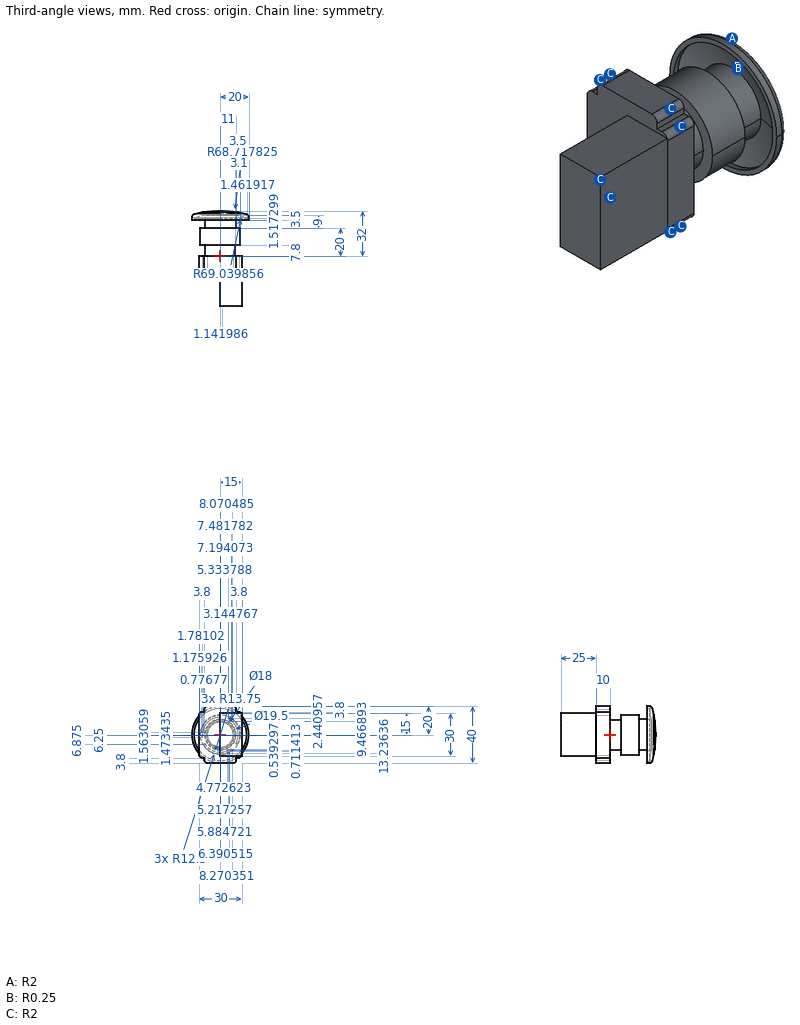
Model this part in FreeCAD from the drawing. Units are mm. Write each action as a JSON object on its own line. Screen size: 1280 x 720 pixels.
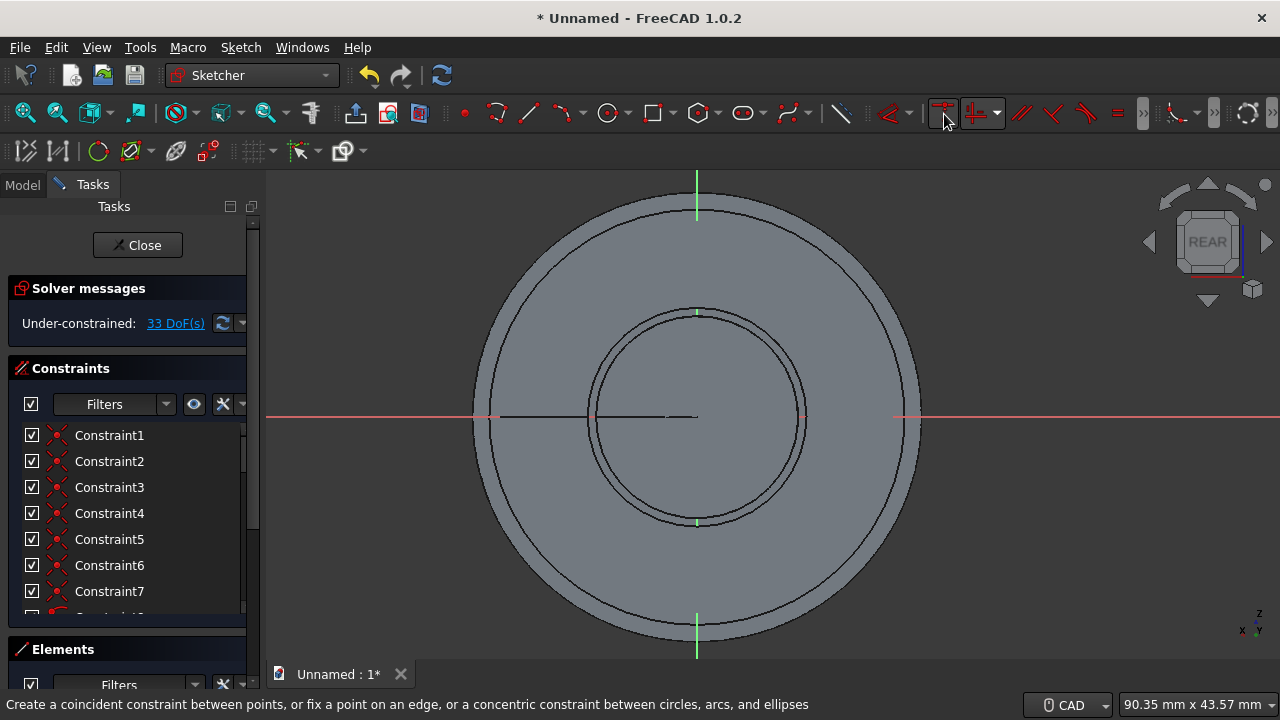
{"action": "left_click_drag", "start_coordinate": [687, 407], "coordinate": [707, 428]}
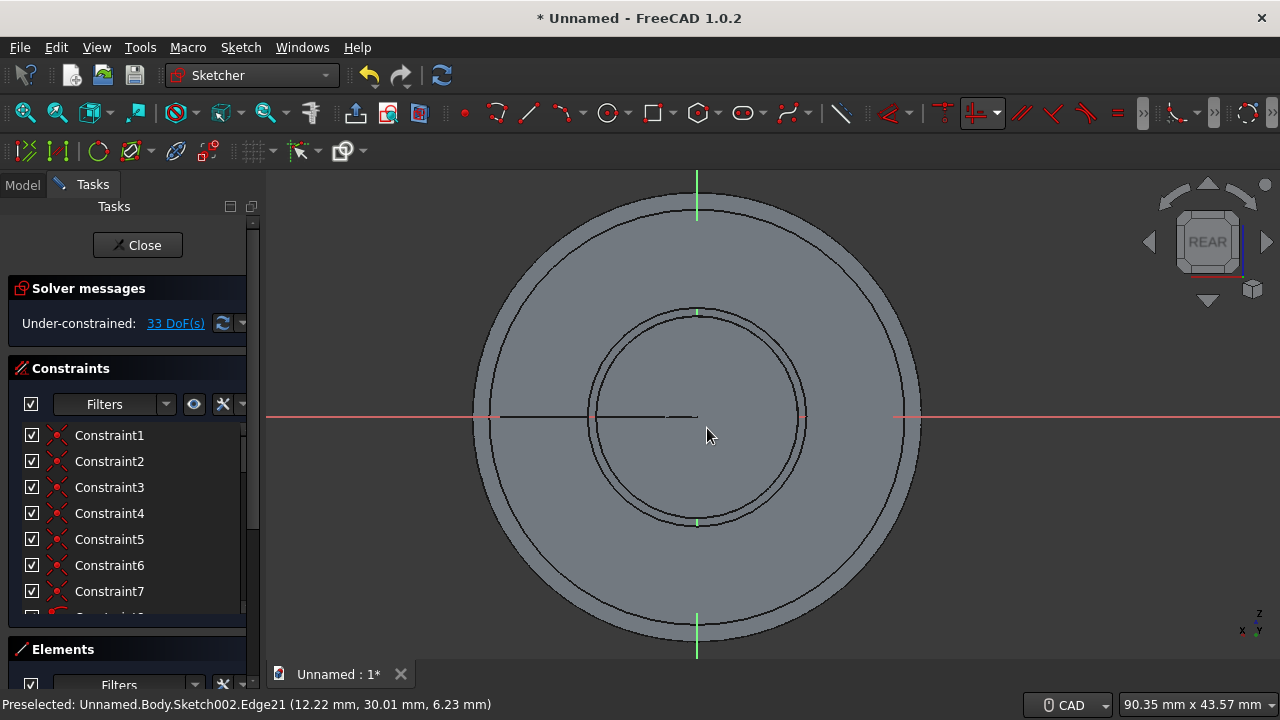
{"action": "left_click", "coordinate": [944, 114]}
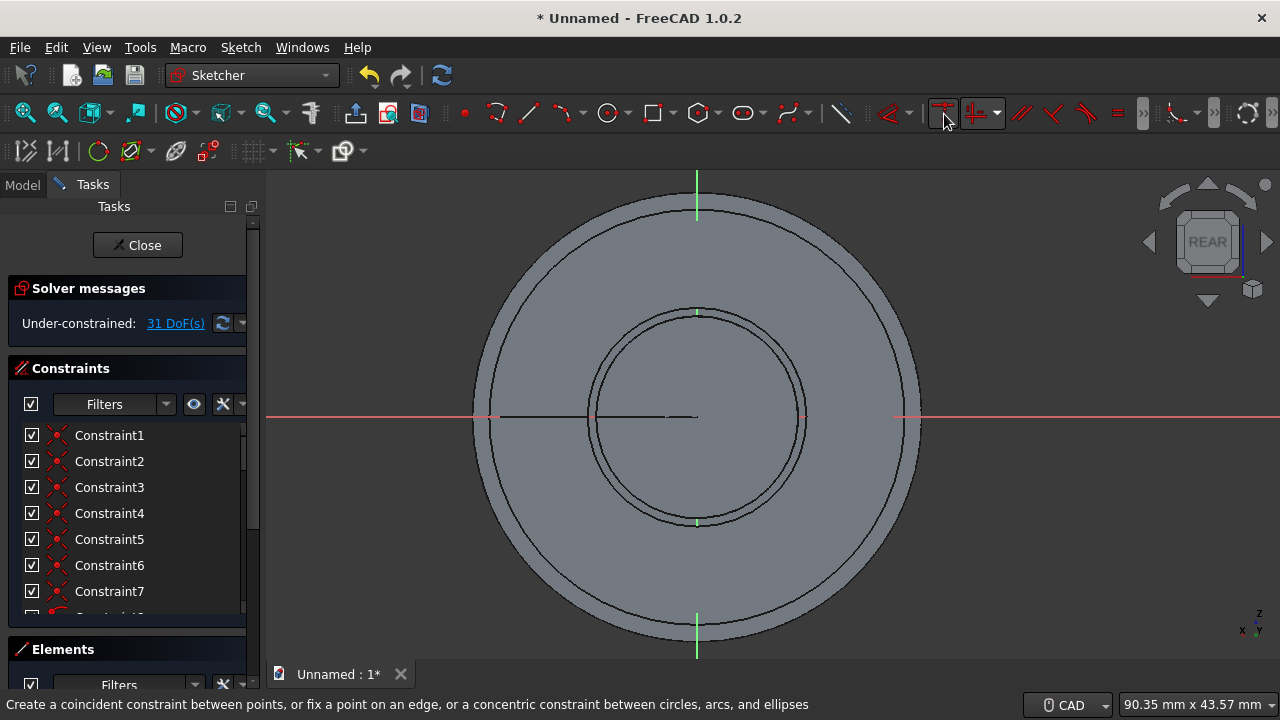
{"action": "left_click", "coordinate": [699, 558]}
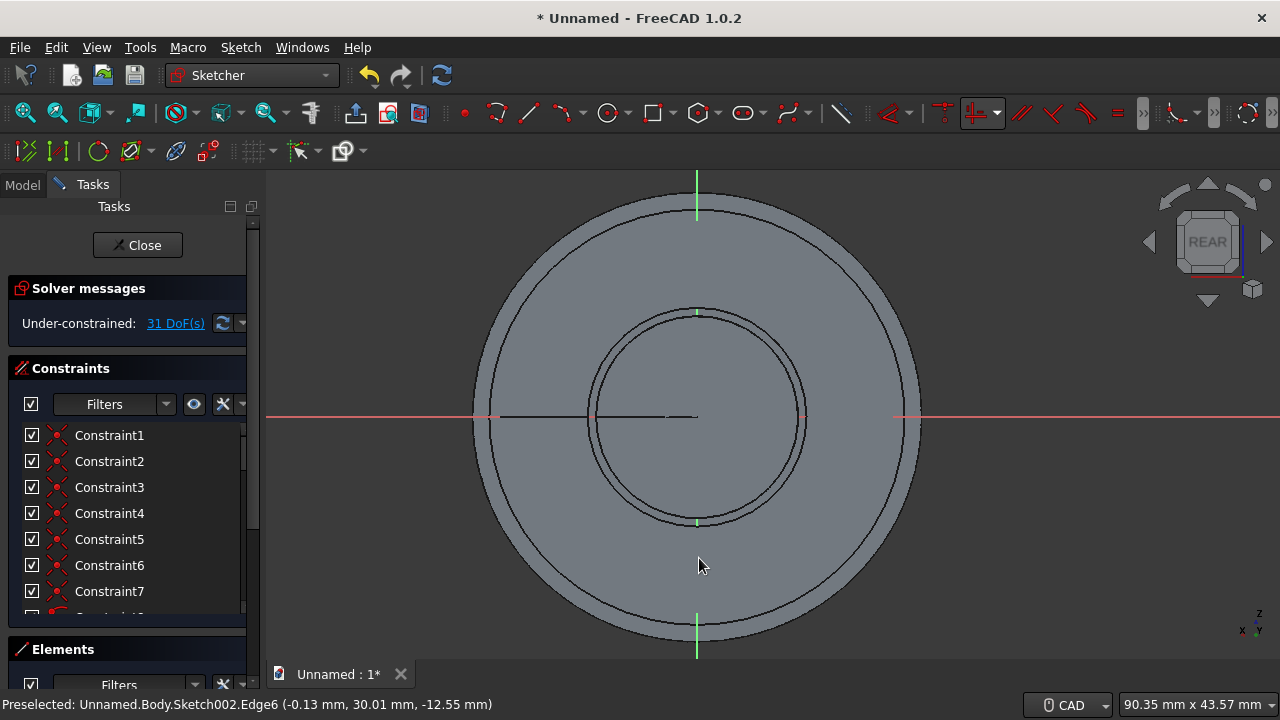
{"action": "left_click", "coordinate": [816, 344]}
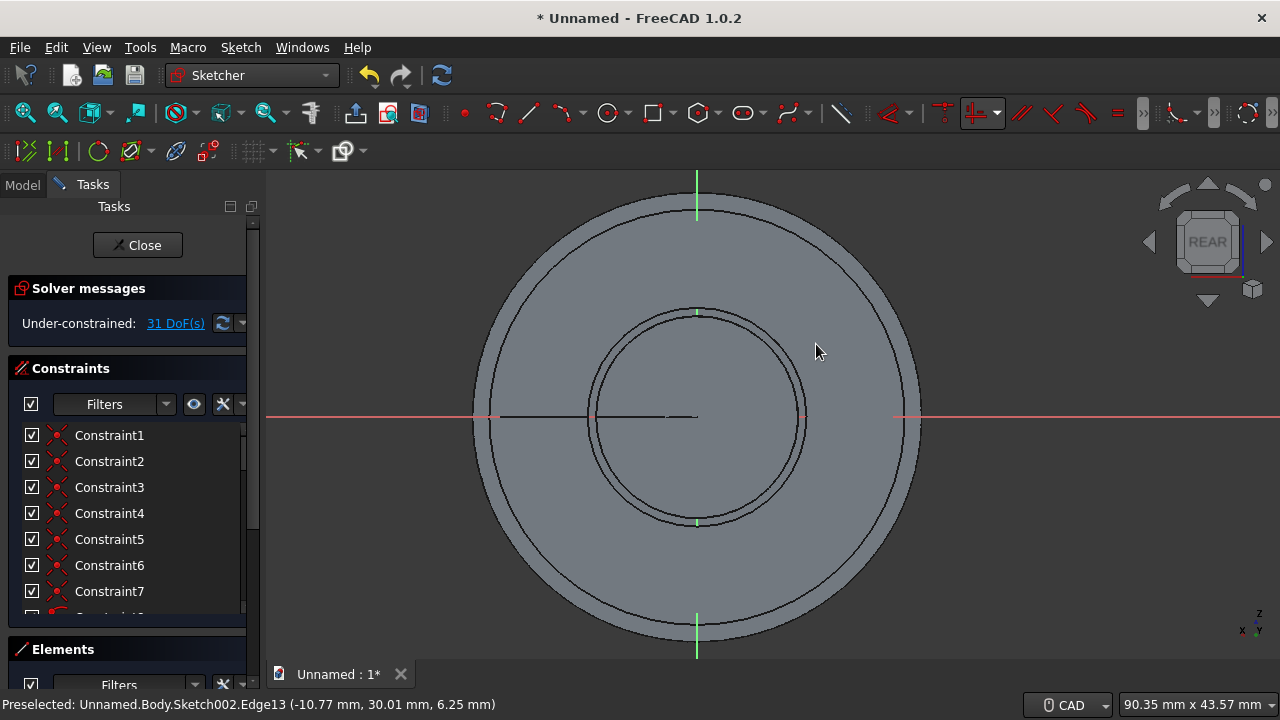
{"action": "left_click", "coordinate": [574, 352]}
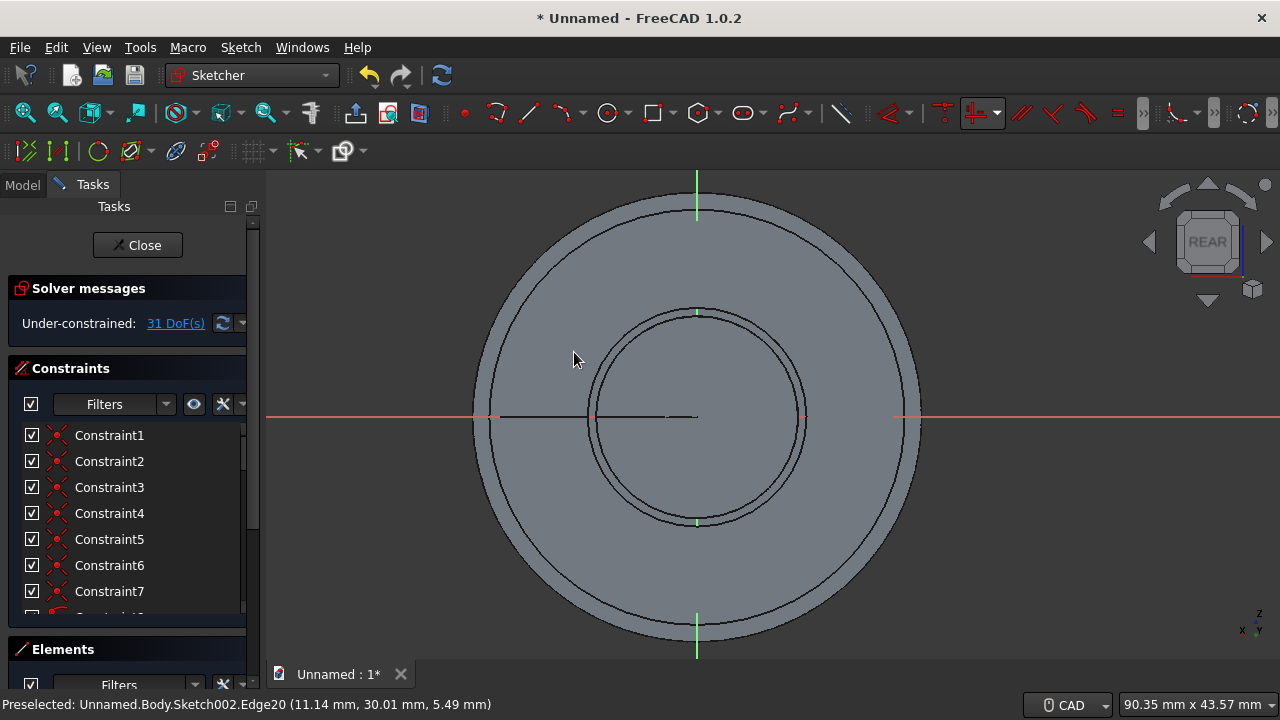
{"action": "left_click", "coordinate": [1118, 114]}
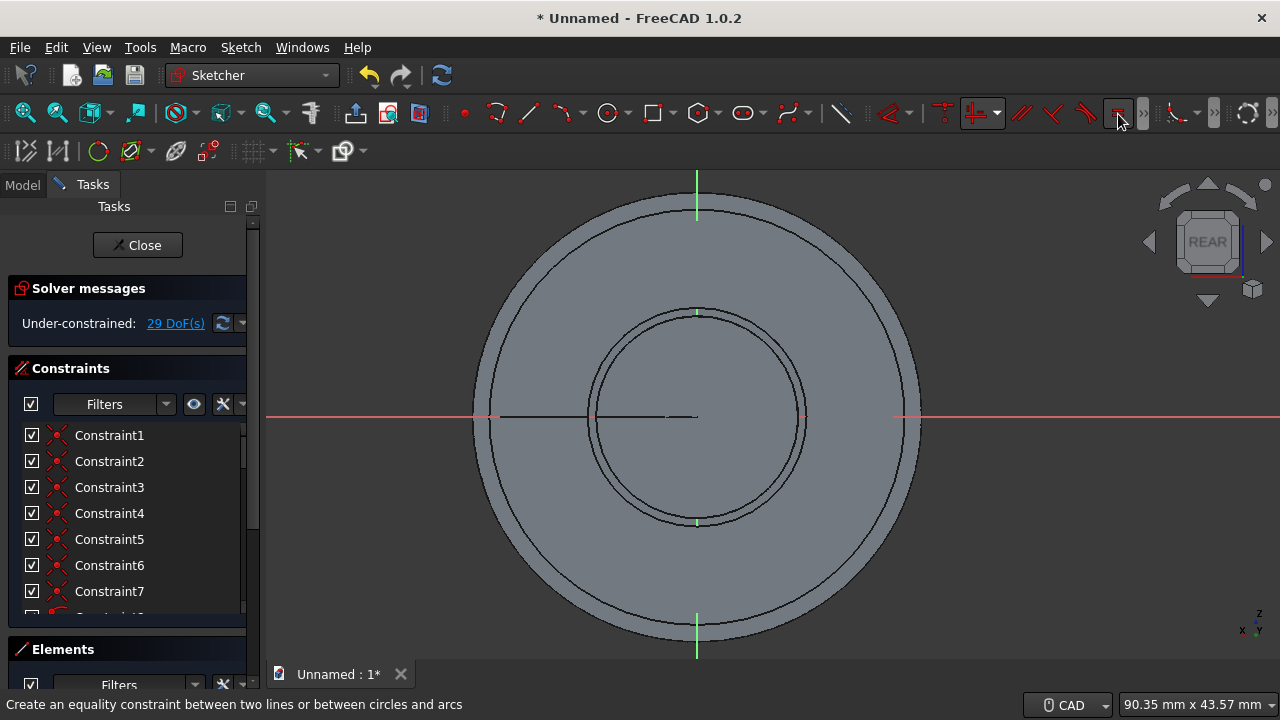
{"action": "left_click", "coordinate": [697, 572]}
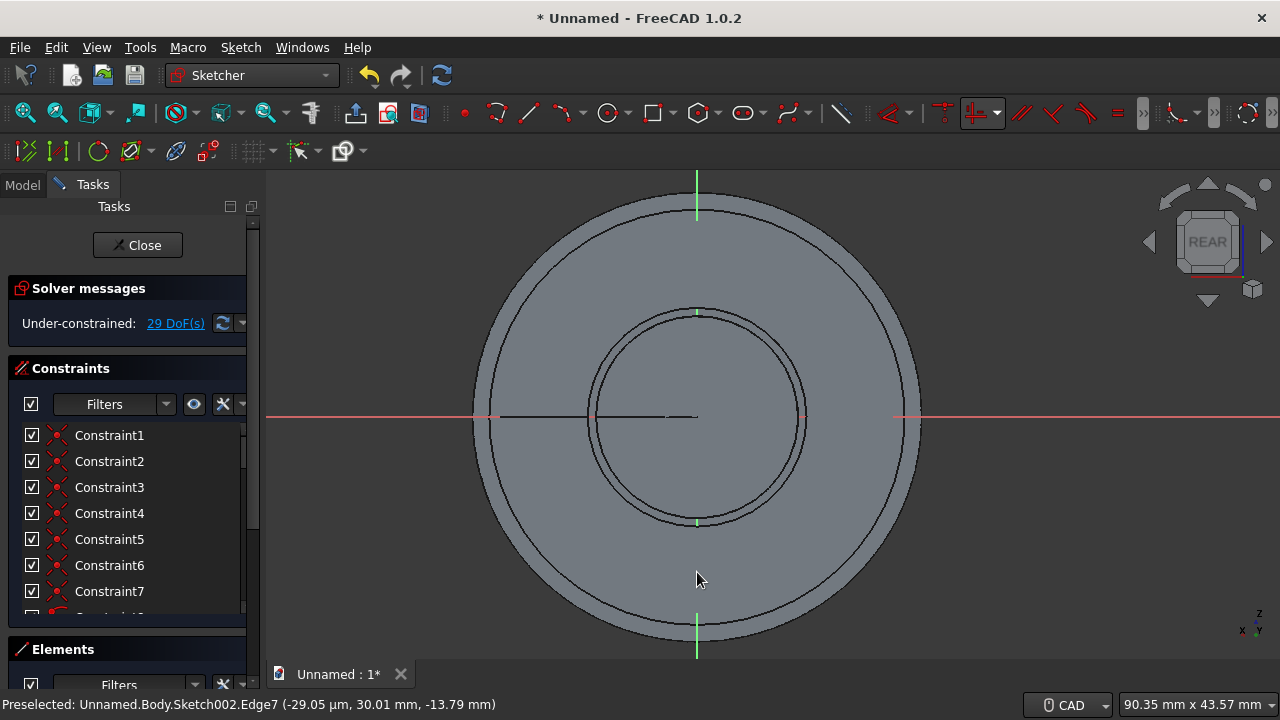
{"action": "left_click", "coordinate": [829, 337]}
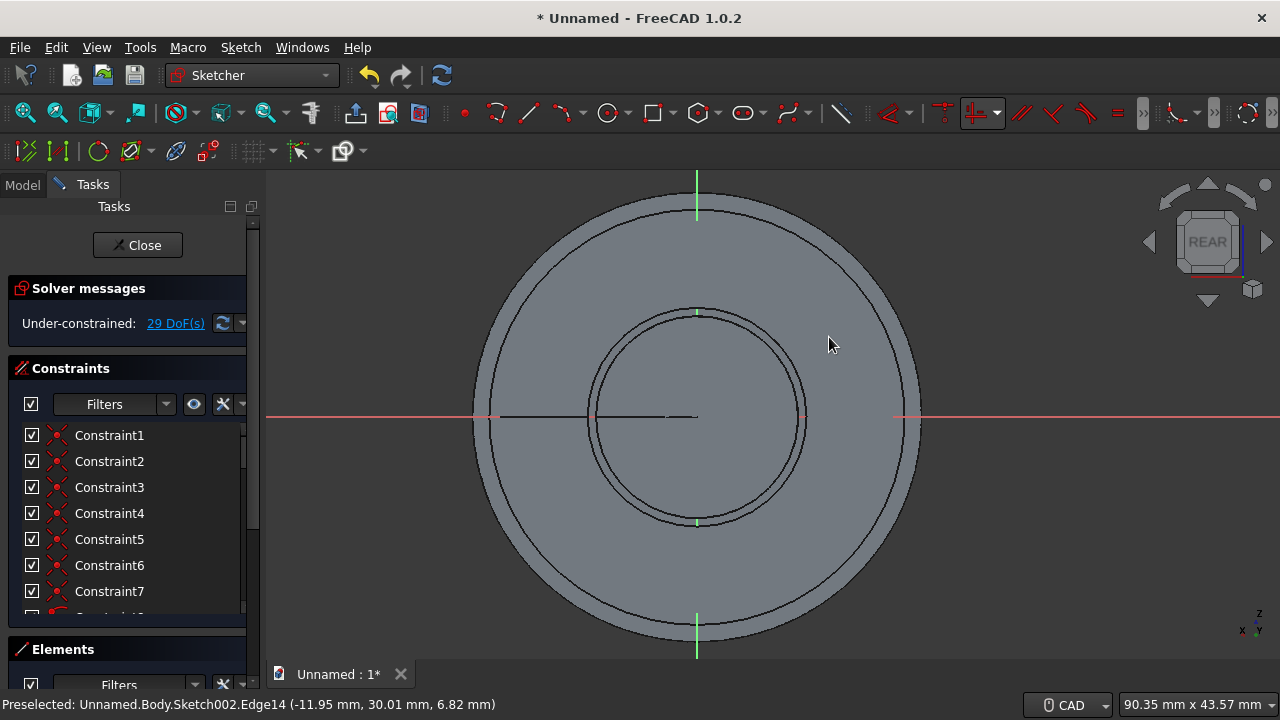
{"action": "left_click", "coordinate": [562, 343]}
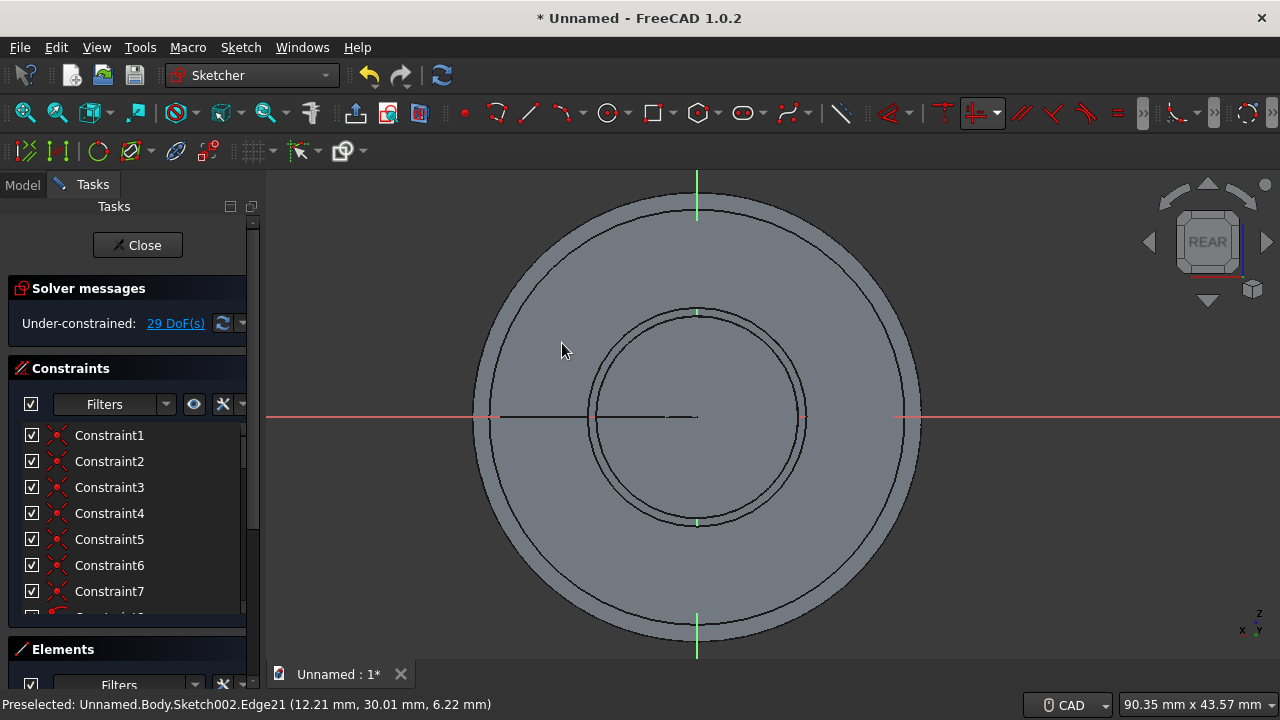
{"action": "left_click", "coordinate": [1118, 114]}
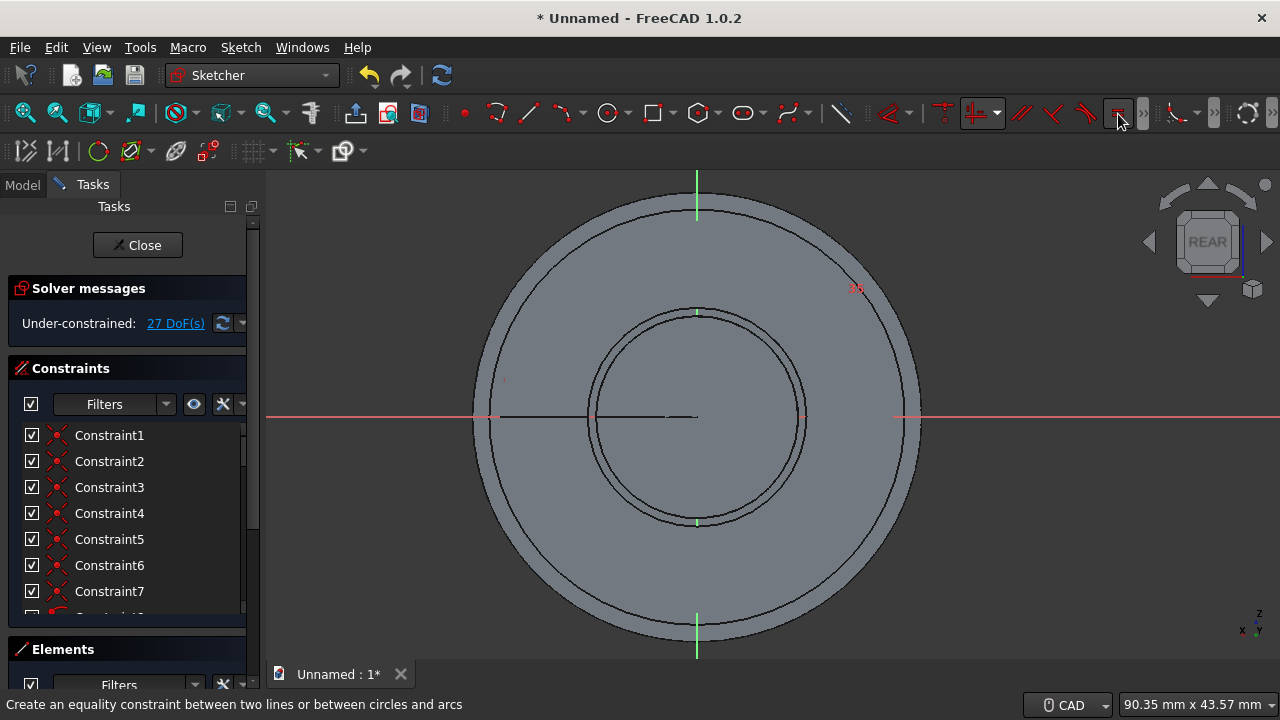
{"action": "left_click", "coordinate": [888, 114]}